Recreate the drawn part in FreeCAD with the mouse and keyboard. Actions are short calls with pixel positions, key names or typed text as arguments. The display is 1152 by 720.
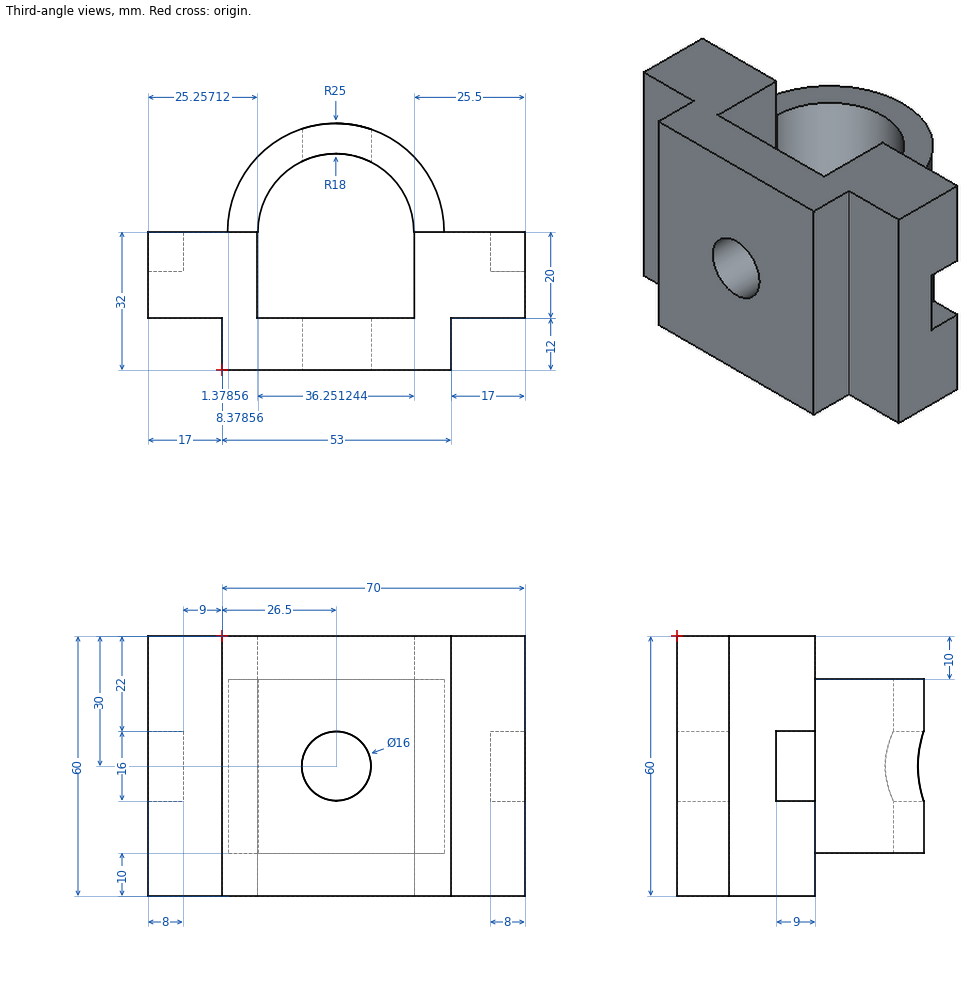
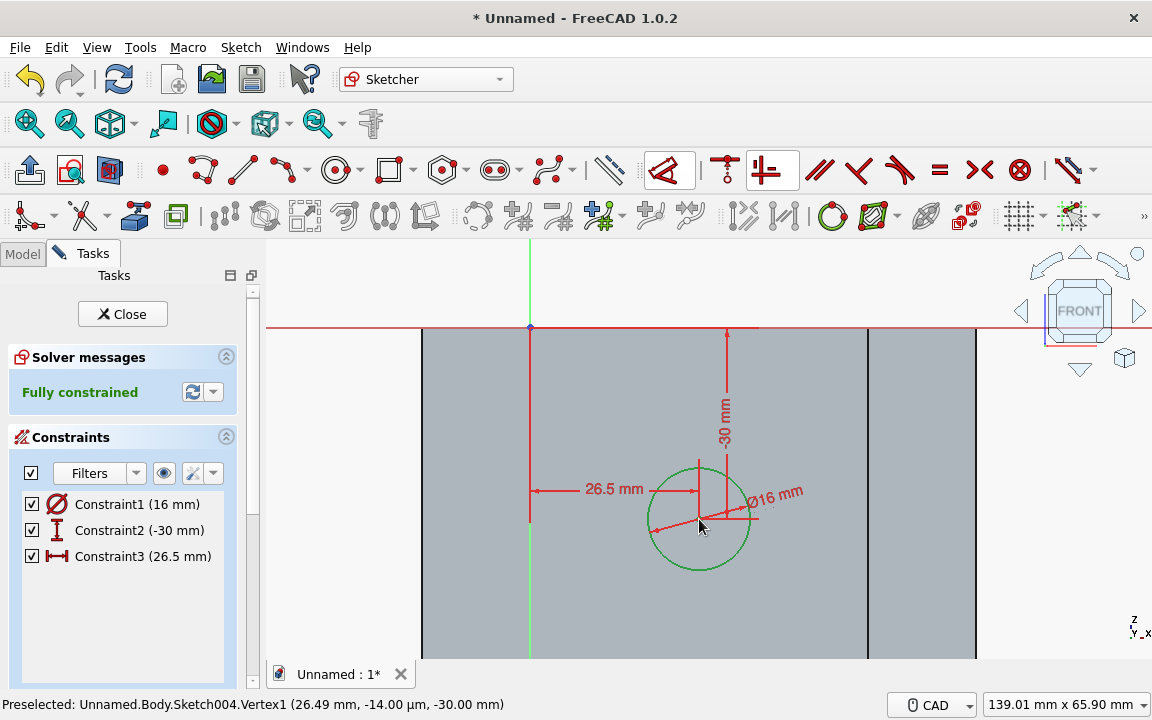
click(123, 314)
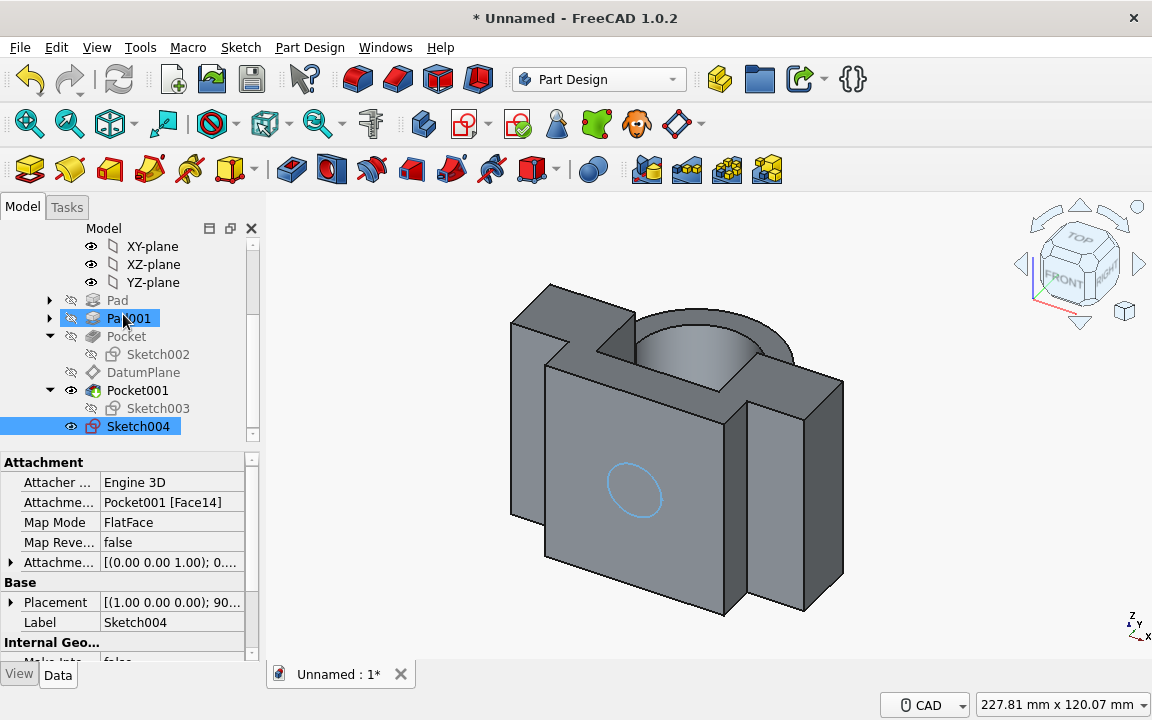
click(292, 170)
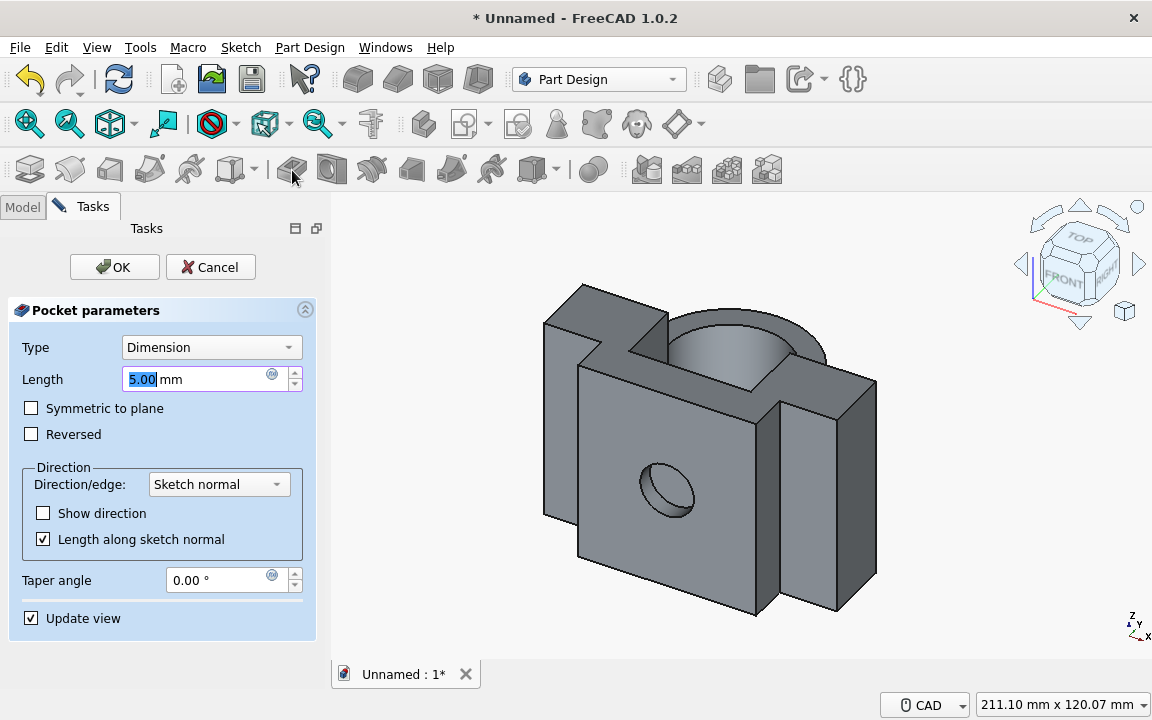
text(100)
key(Tab)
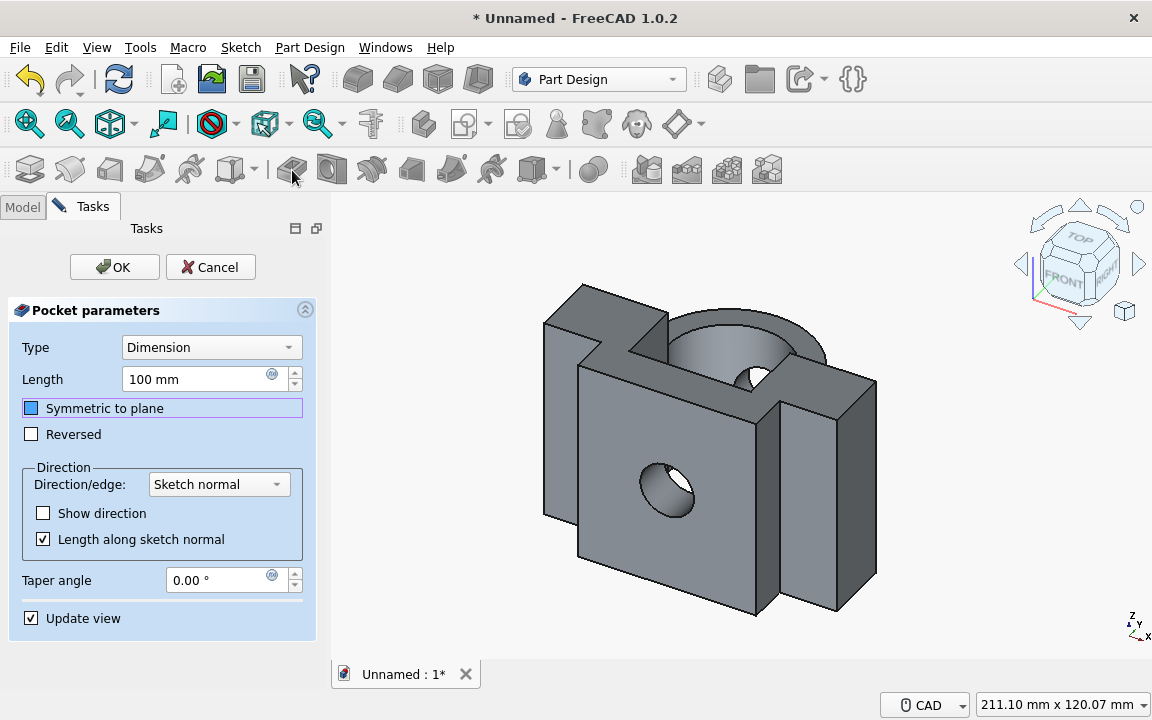
click(115, 267)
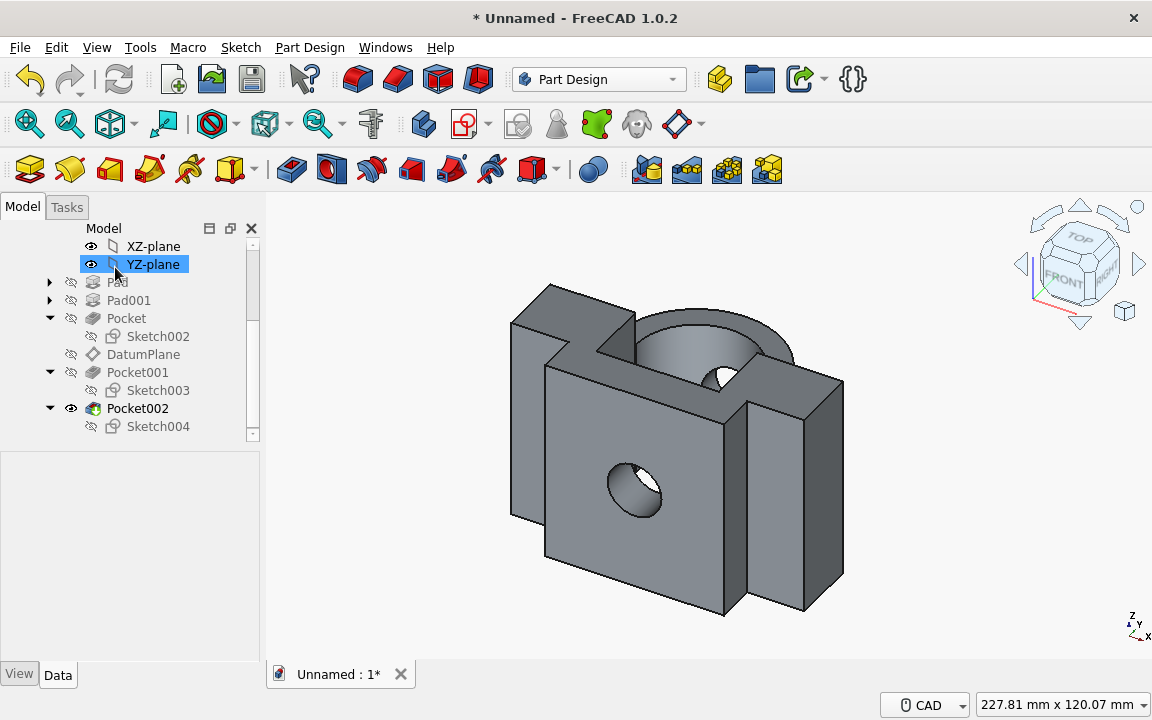
key(4)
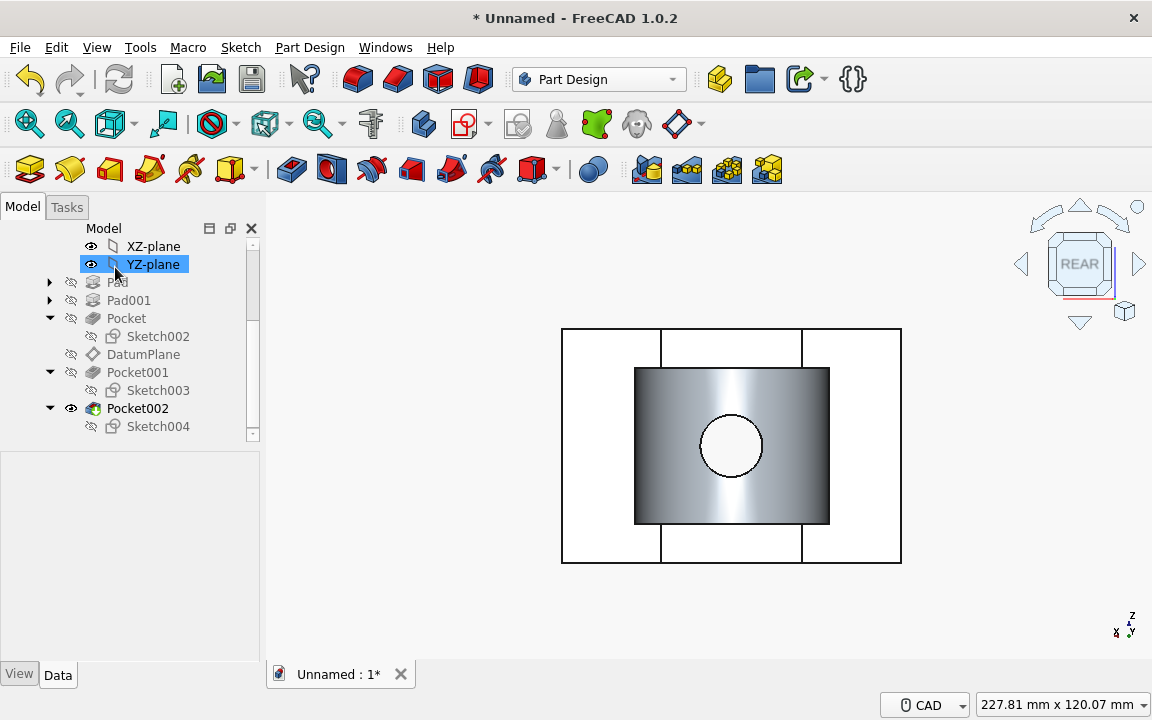
click(598, 378)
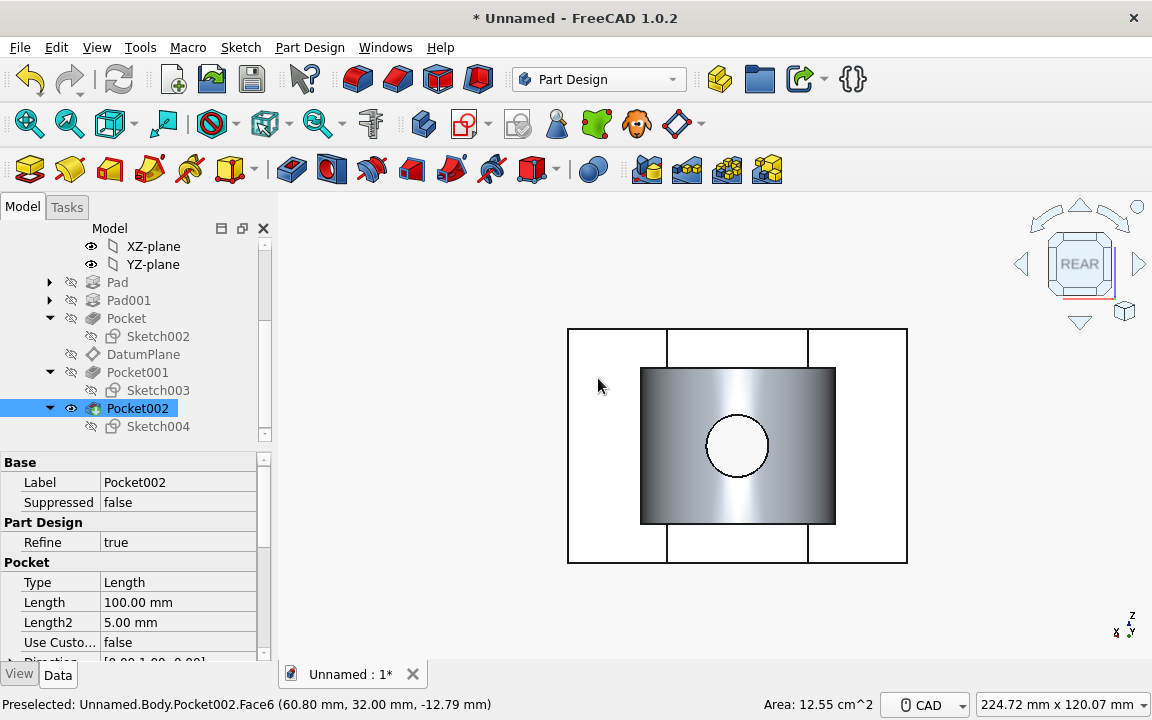
click(464, 124)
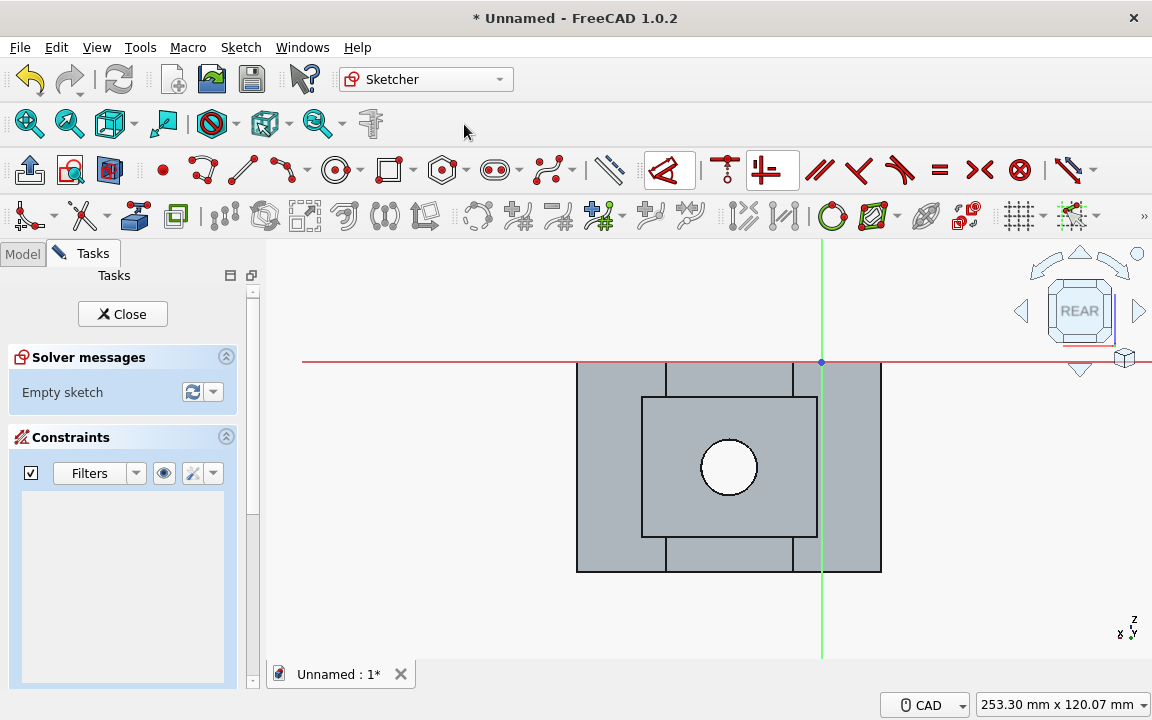
key(q)
key(s)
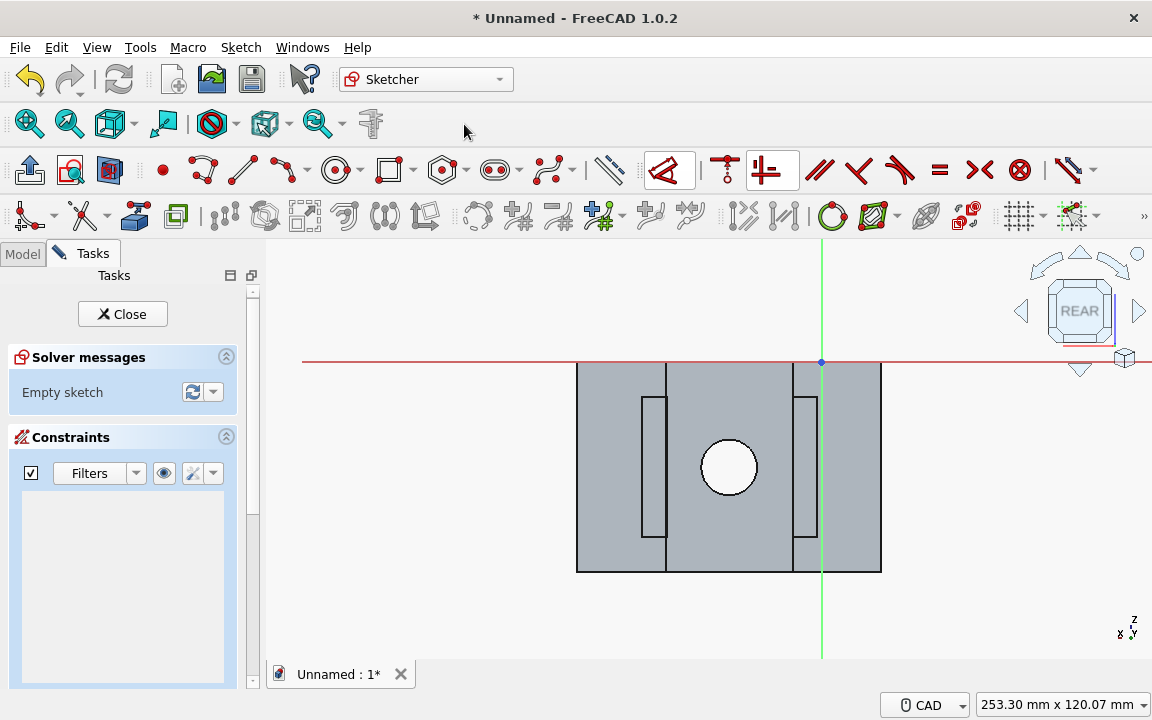
scroll(909, 388, up, 2)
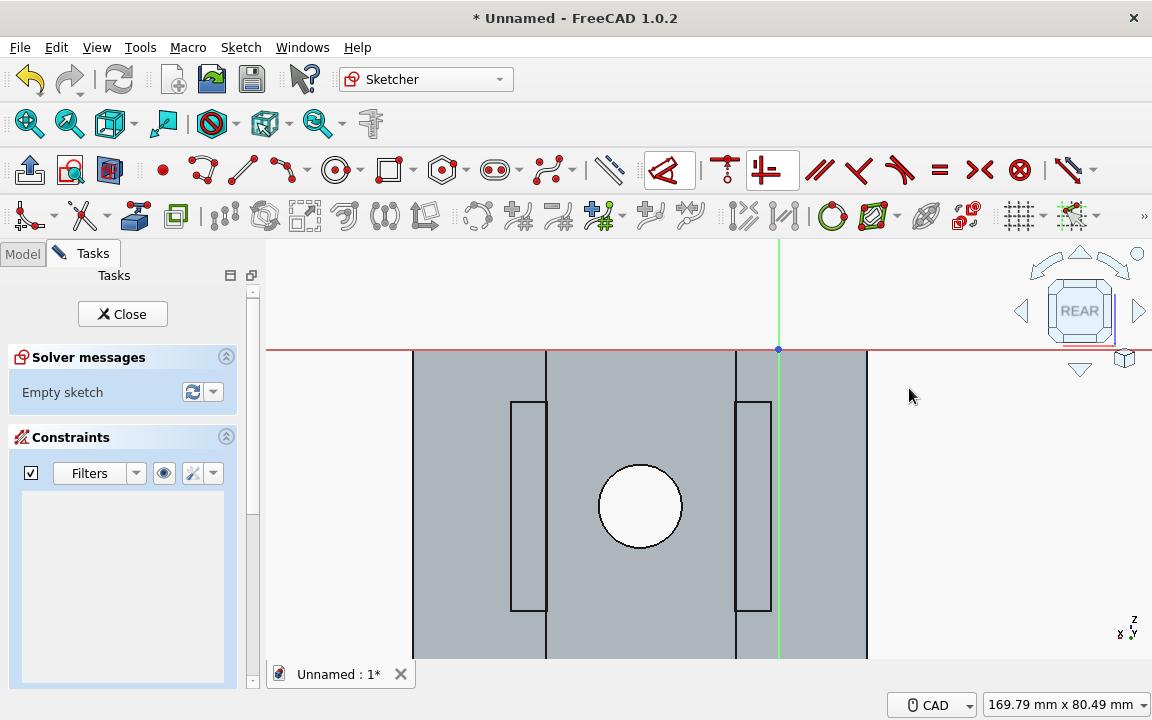
key(g)
key(r)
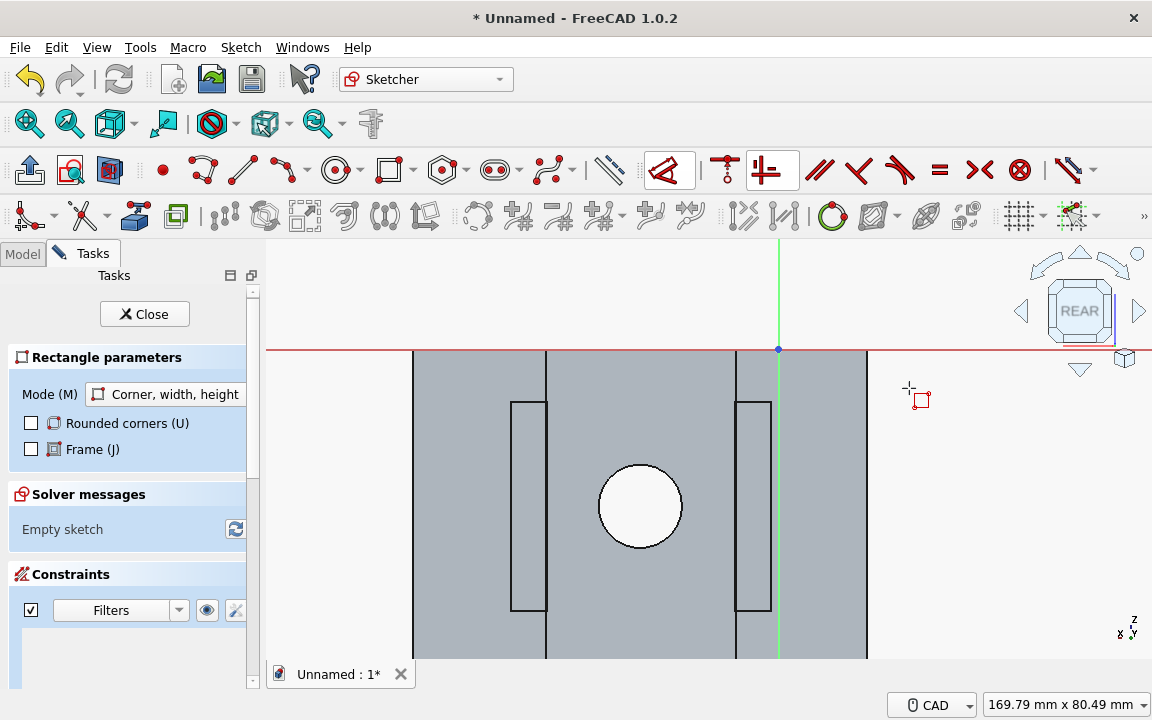
click(826, 465)
click(867, 548)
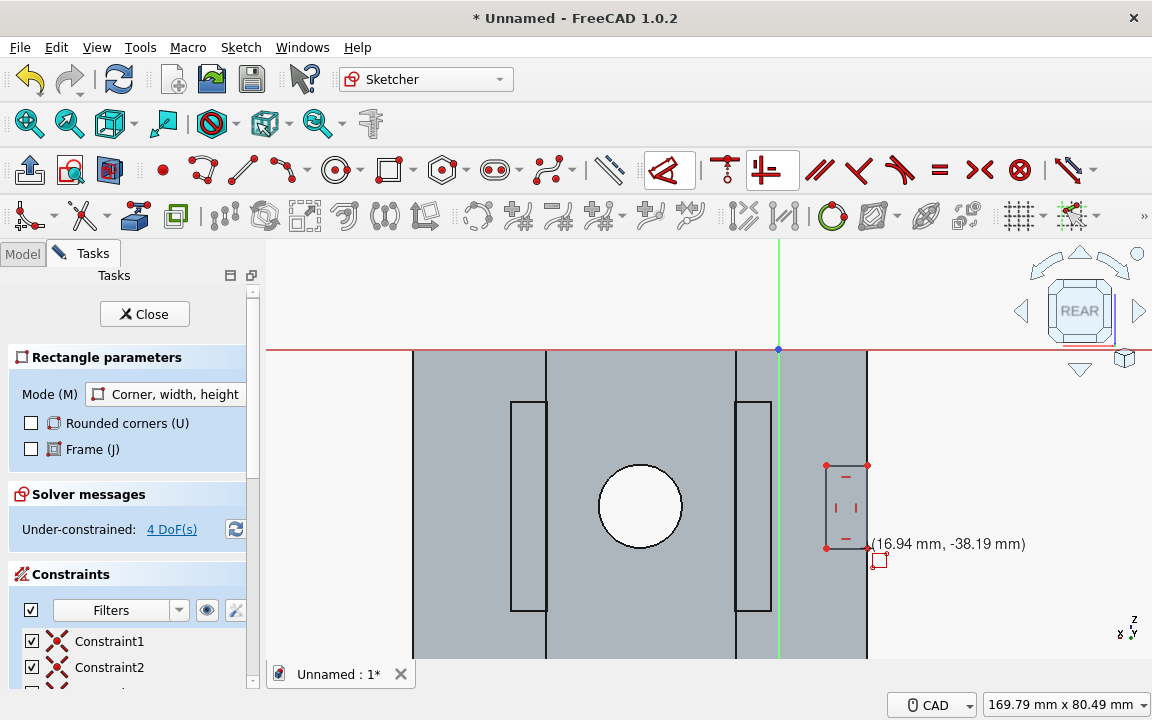
click(413, 465)
click(455, 548)
key(Escape)